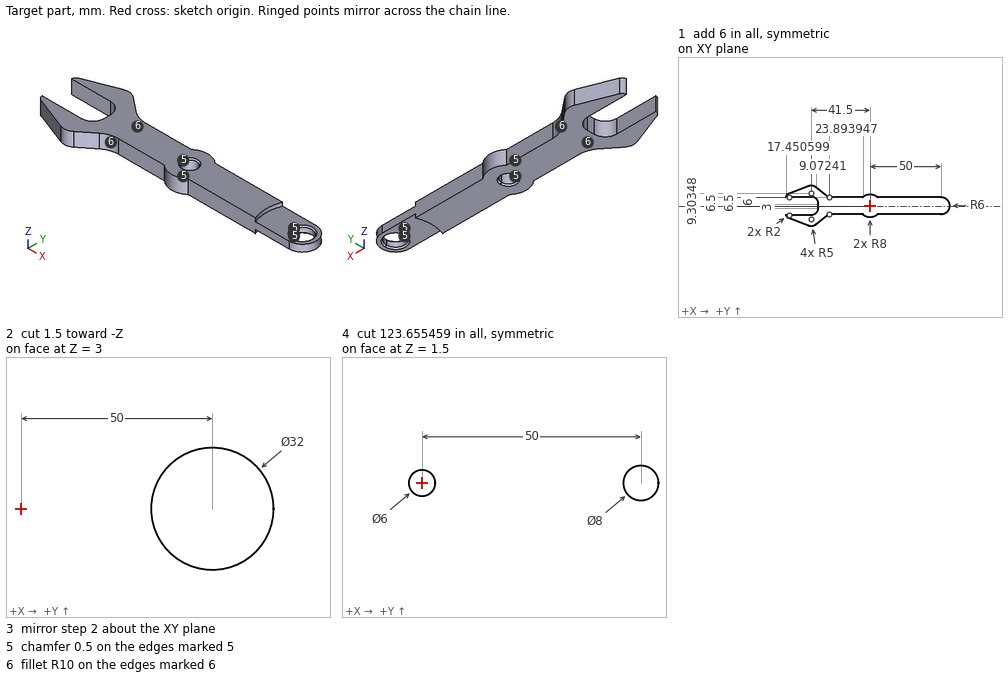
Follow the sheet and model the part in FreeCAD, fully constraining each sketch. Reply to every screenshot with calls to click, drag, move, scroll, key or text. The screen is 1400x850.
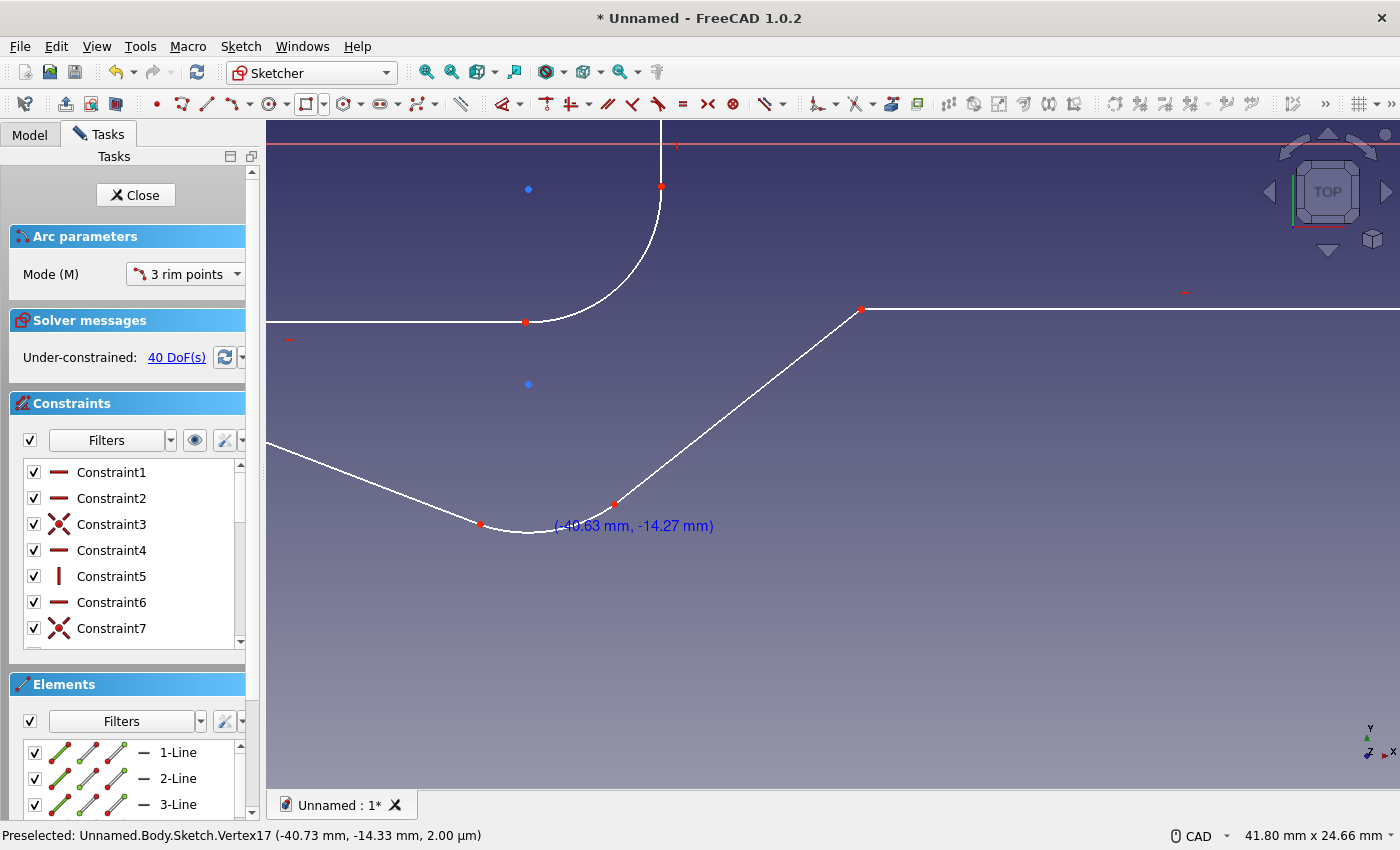
scroll(550, 533, down, 8)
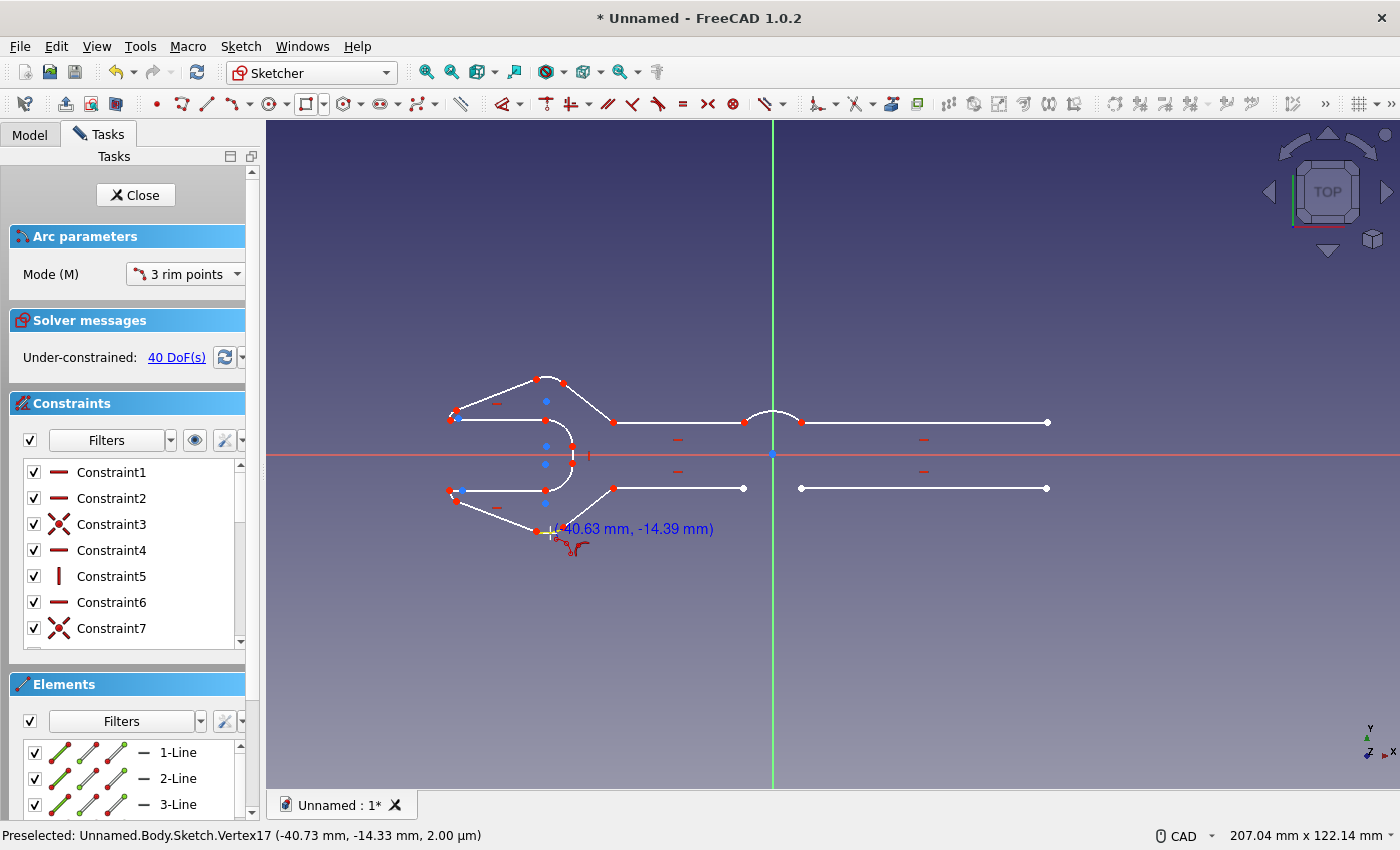
click(744, 488)
click(802, 488)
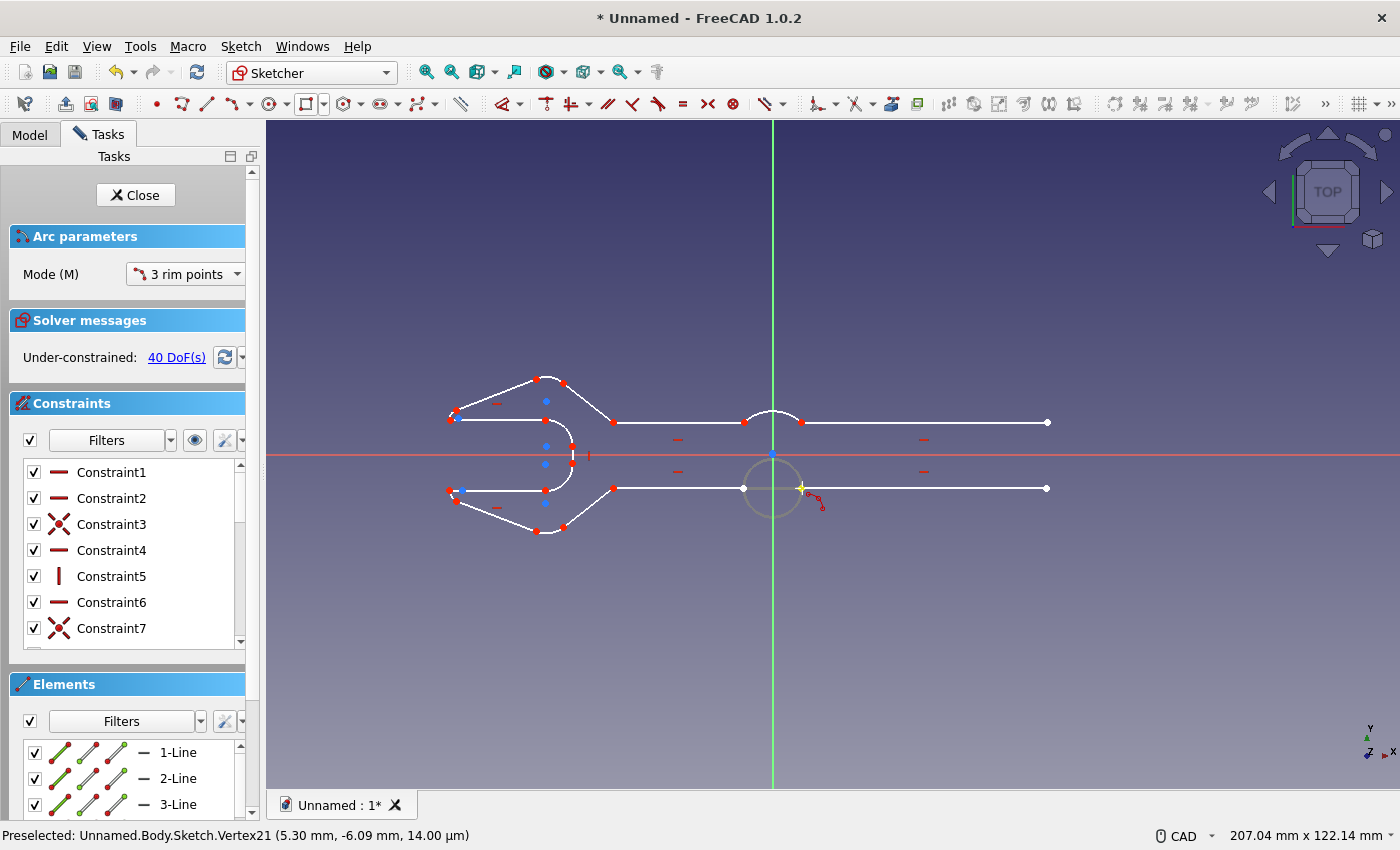
scroll(760, 497, up, 3)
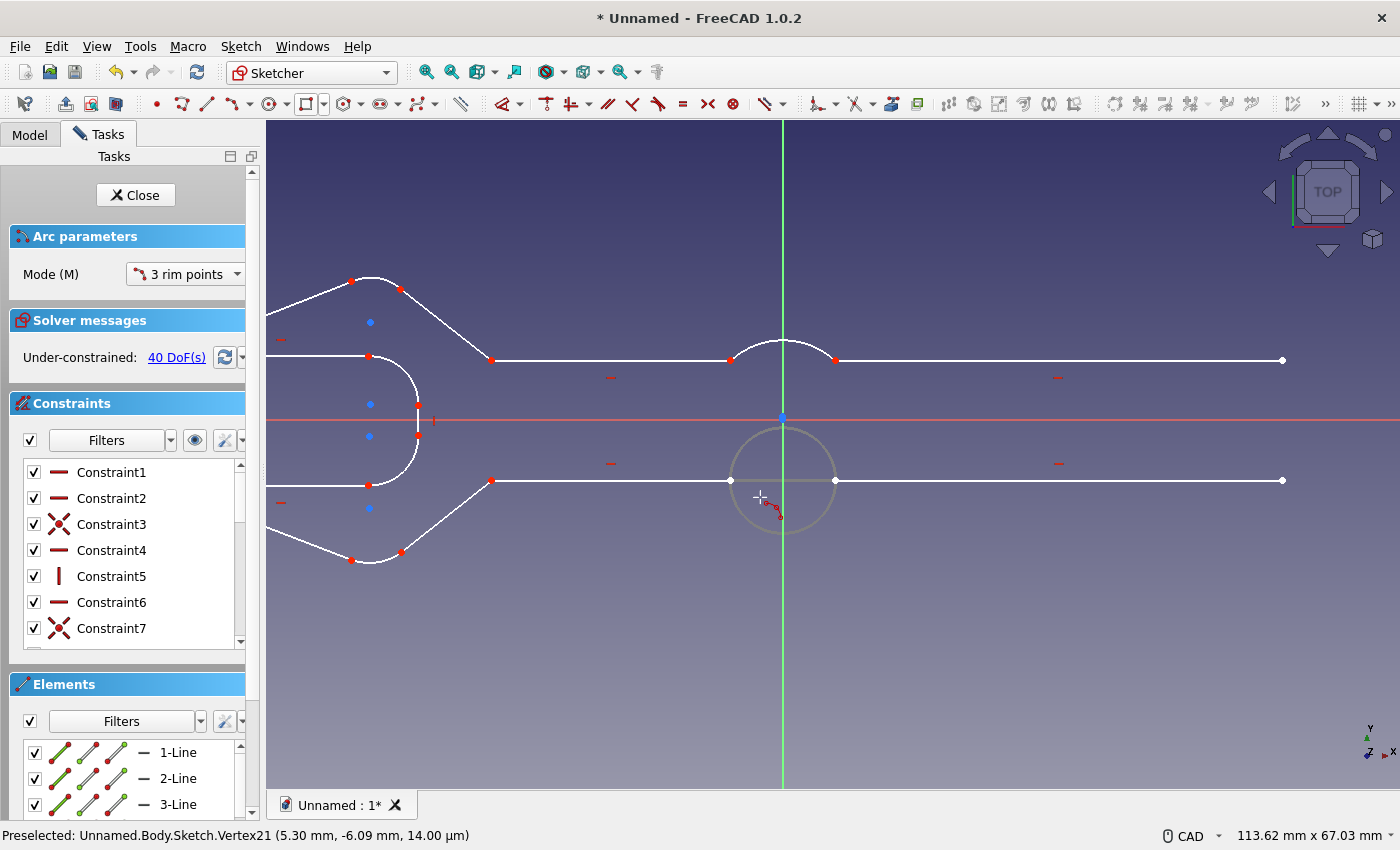
click(760, 496)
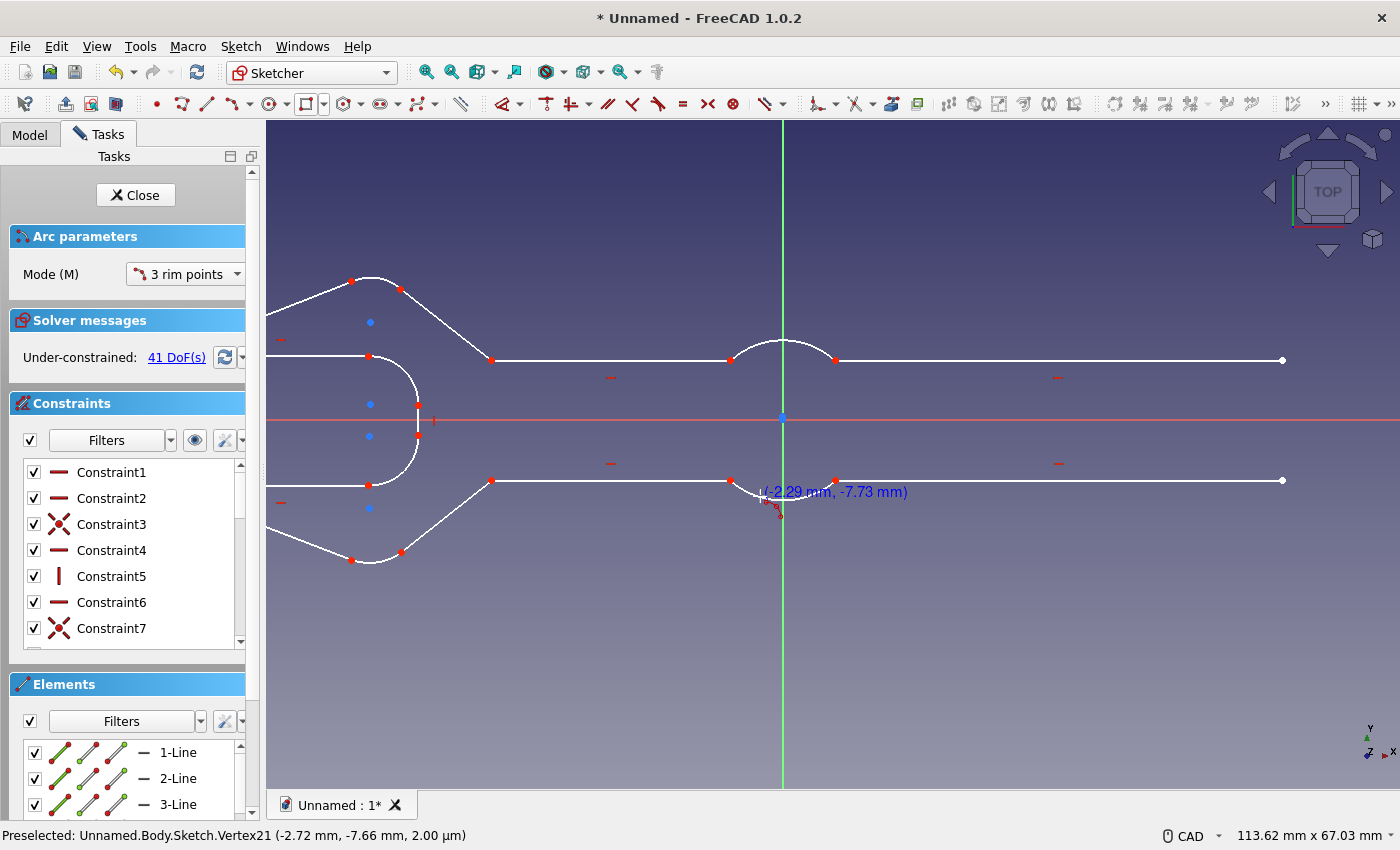
scroll(760, 497, down, 3)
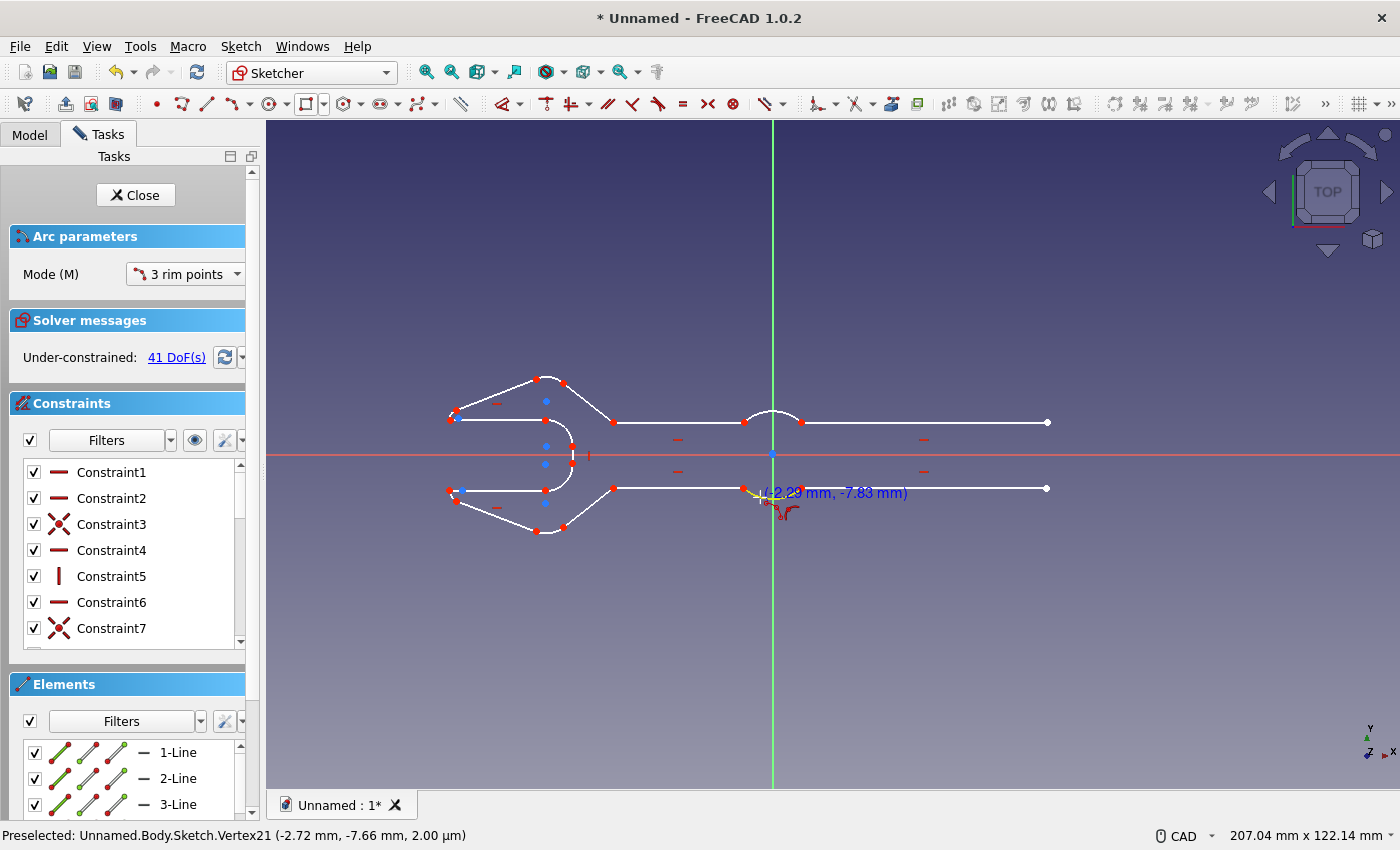
click(1047, 488)
click(1047, 423)
click(1073, 474)
key(Escape)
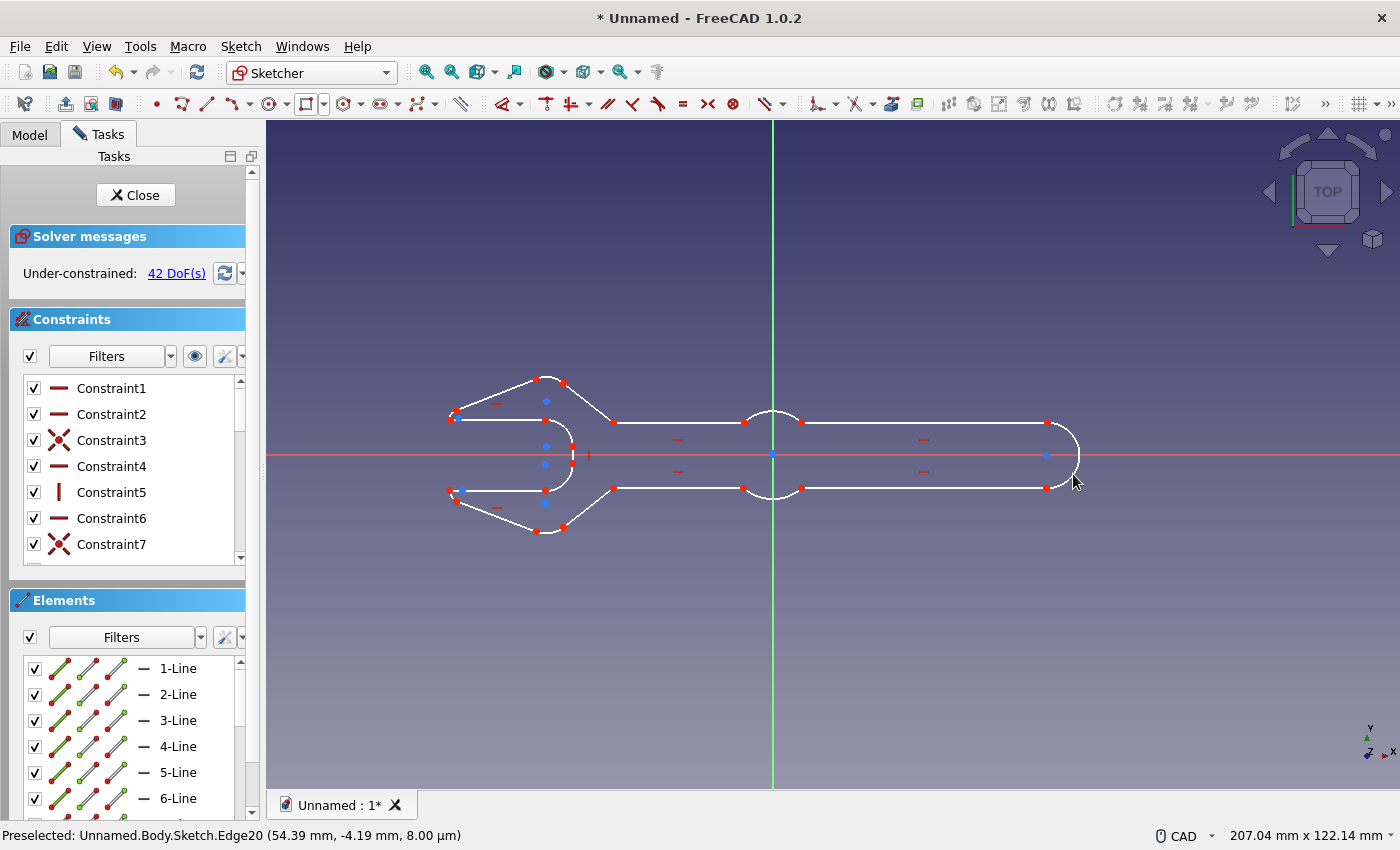
click(973, 423)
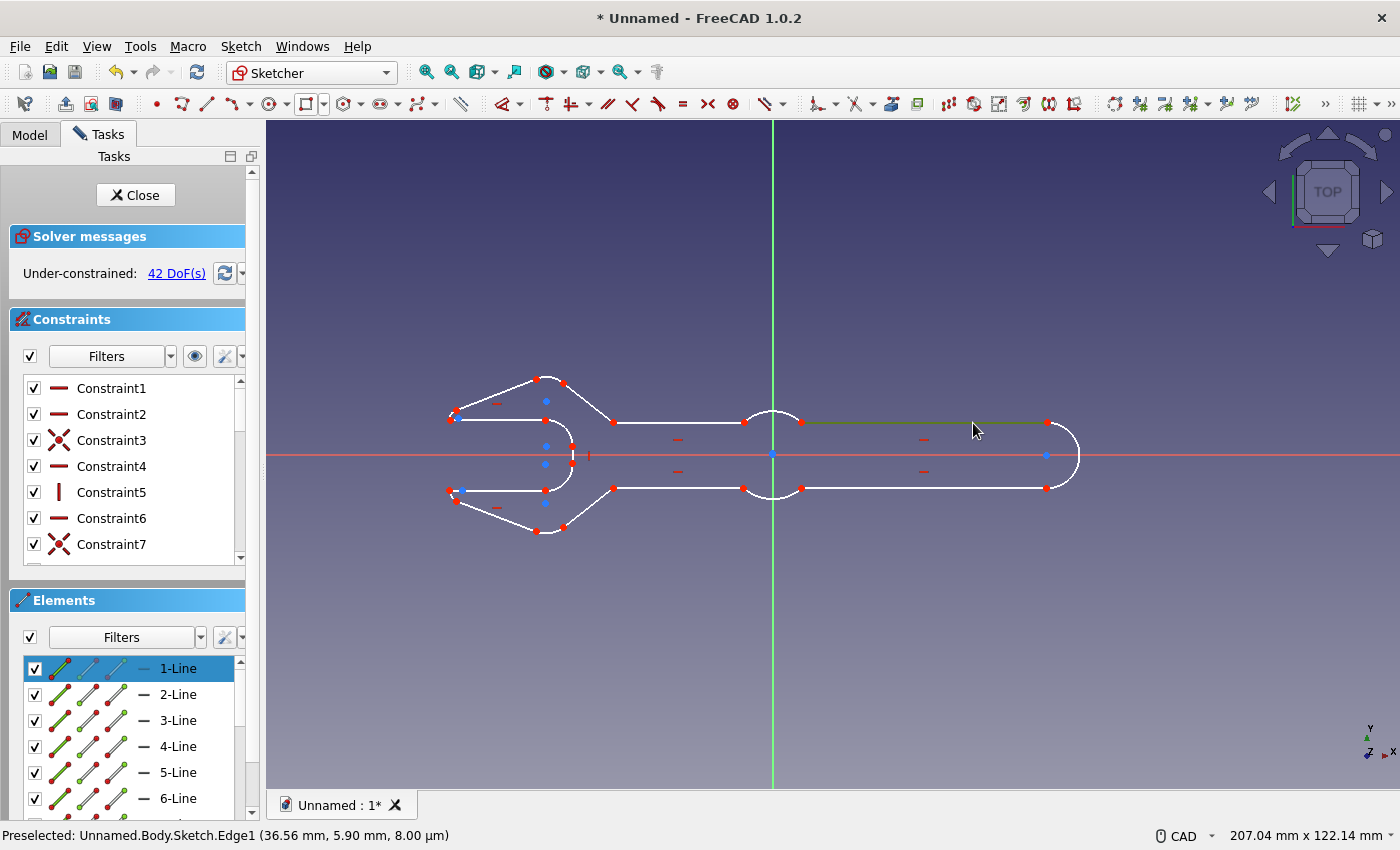
click(1073, 475)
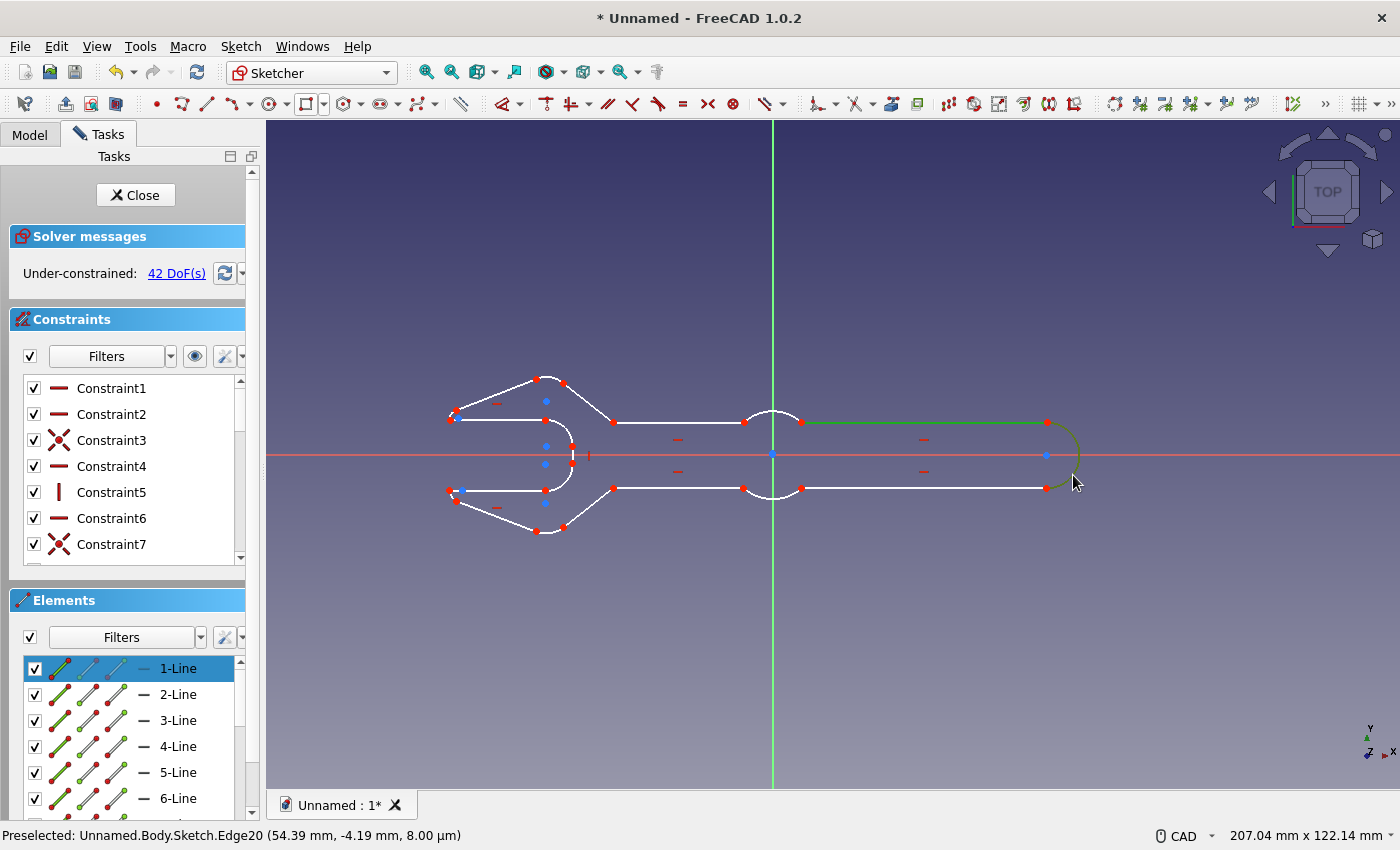
click(658, 104)